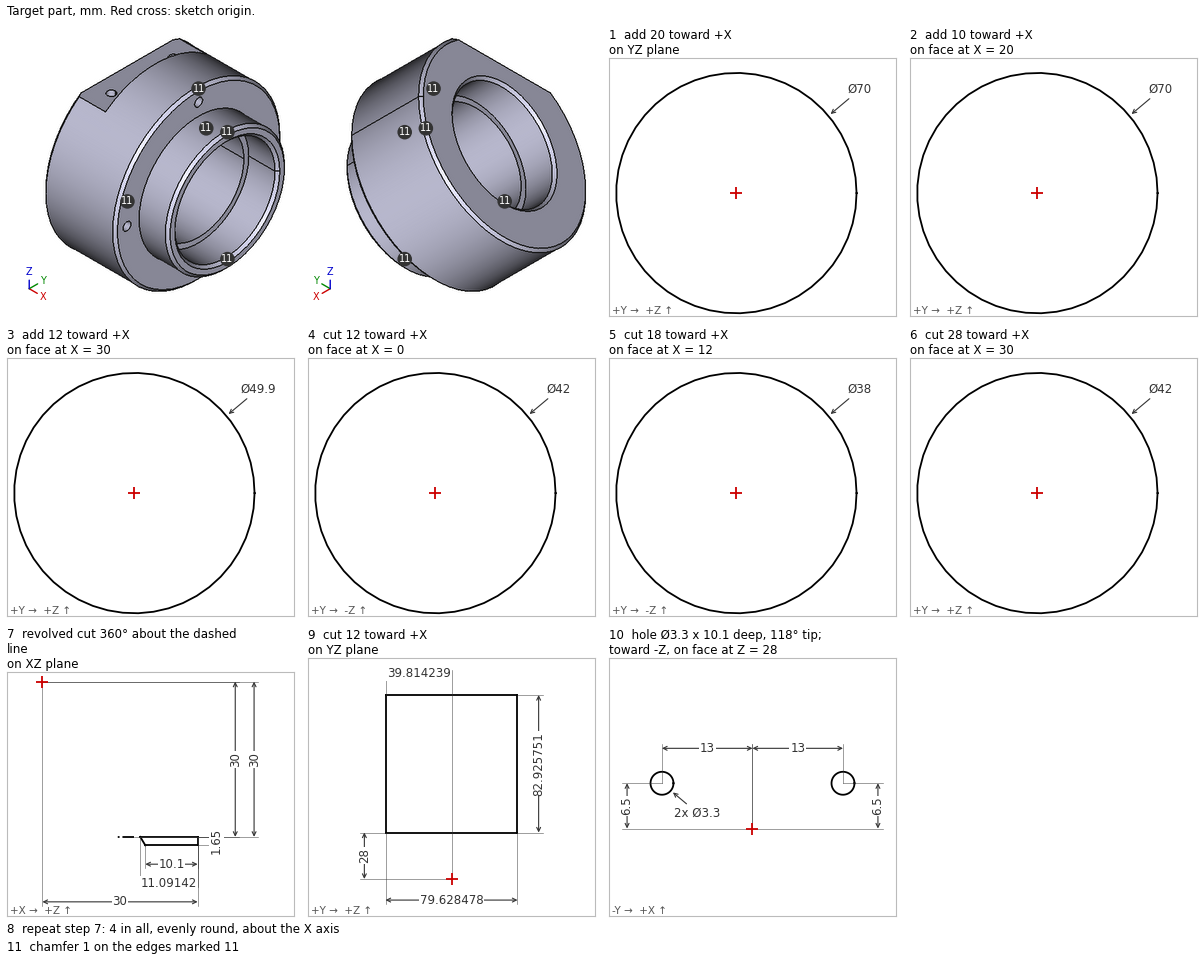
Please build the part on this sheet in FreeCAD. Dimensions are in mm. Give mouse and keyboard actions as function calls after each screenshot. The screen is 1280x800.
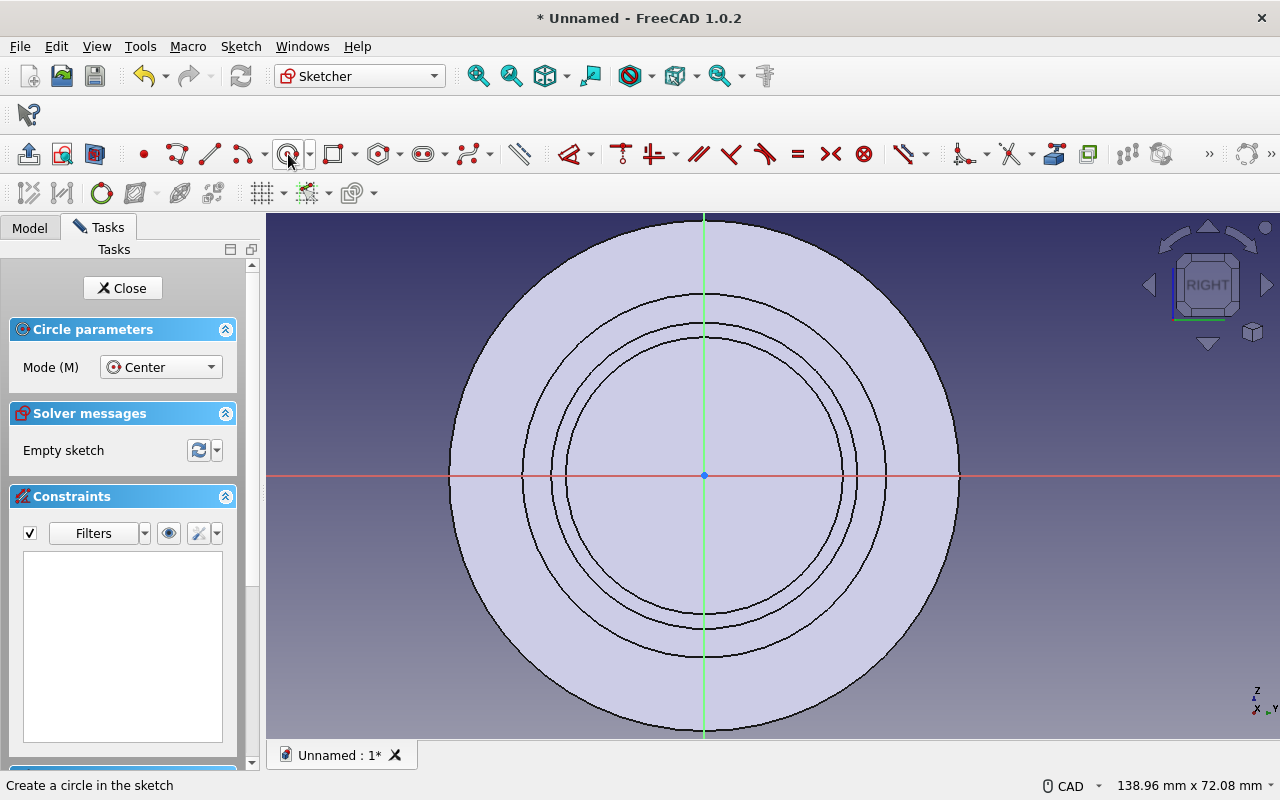
click(704, 476)
move(813, 367)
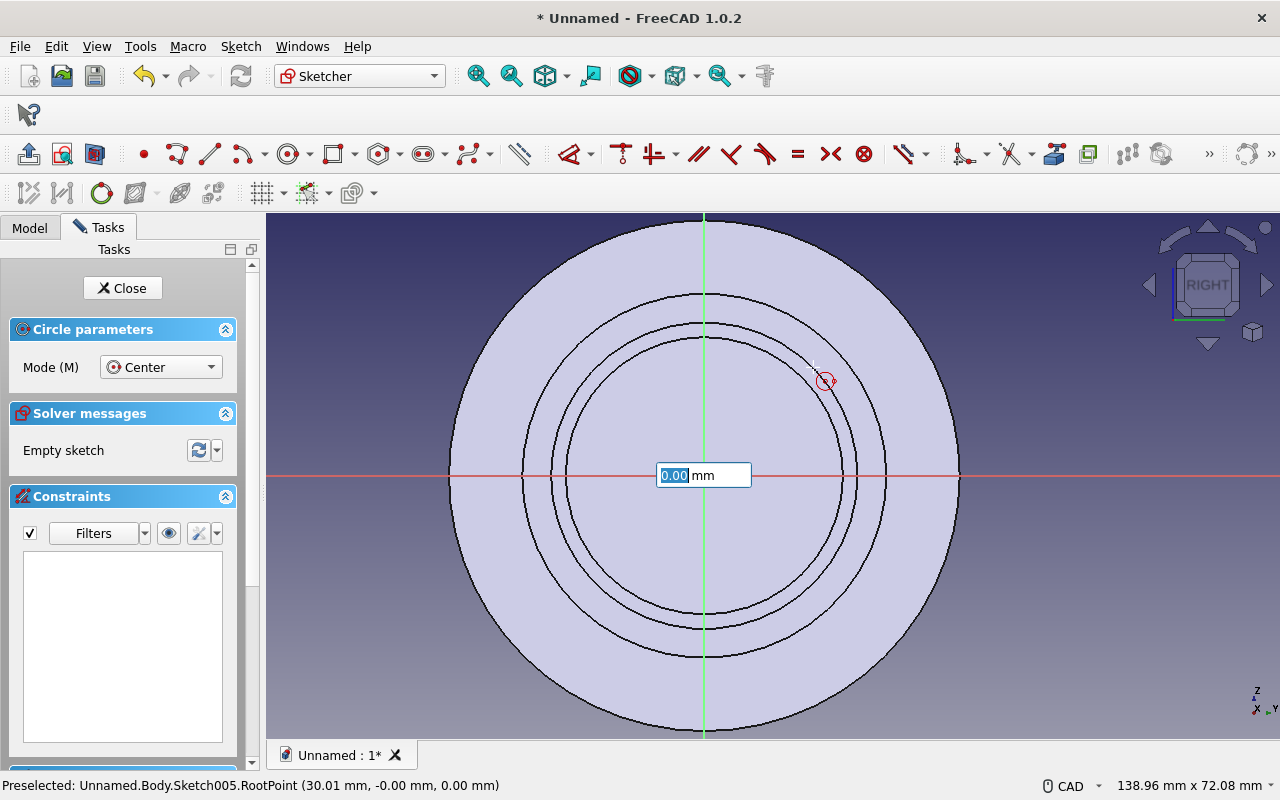
text(42)
key(Return)
key(Escape)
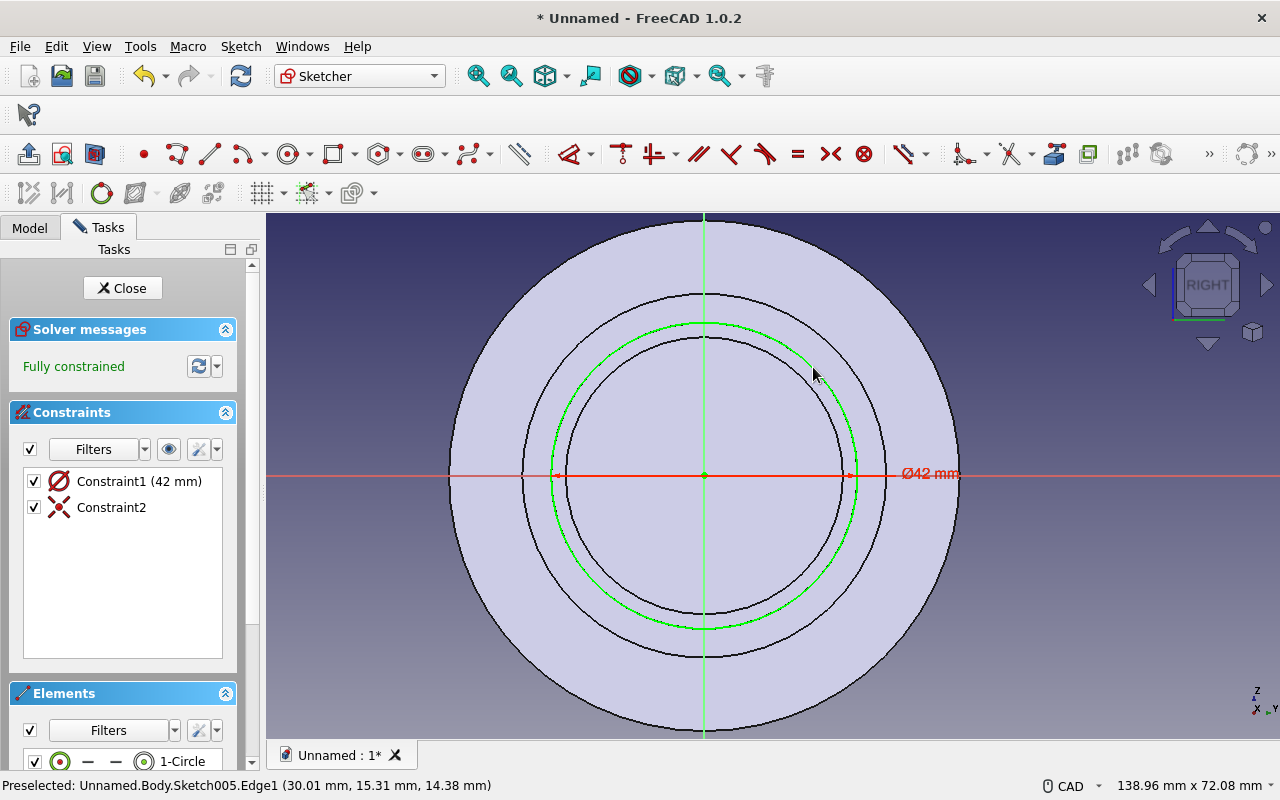
click(123, 288)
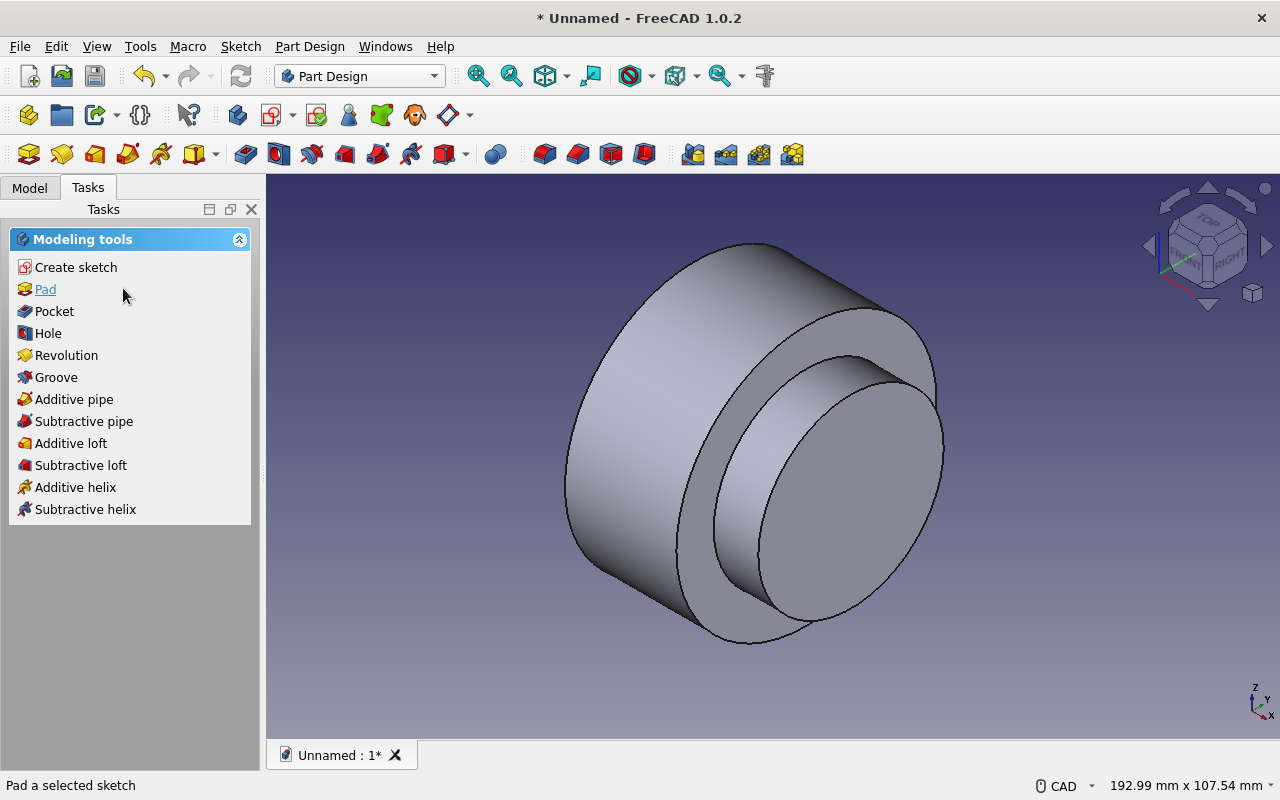
click(246, 154)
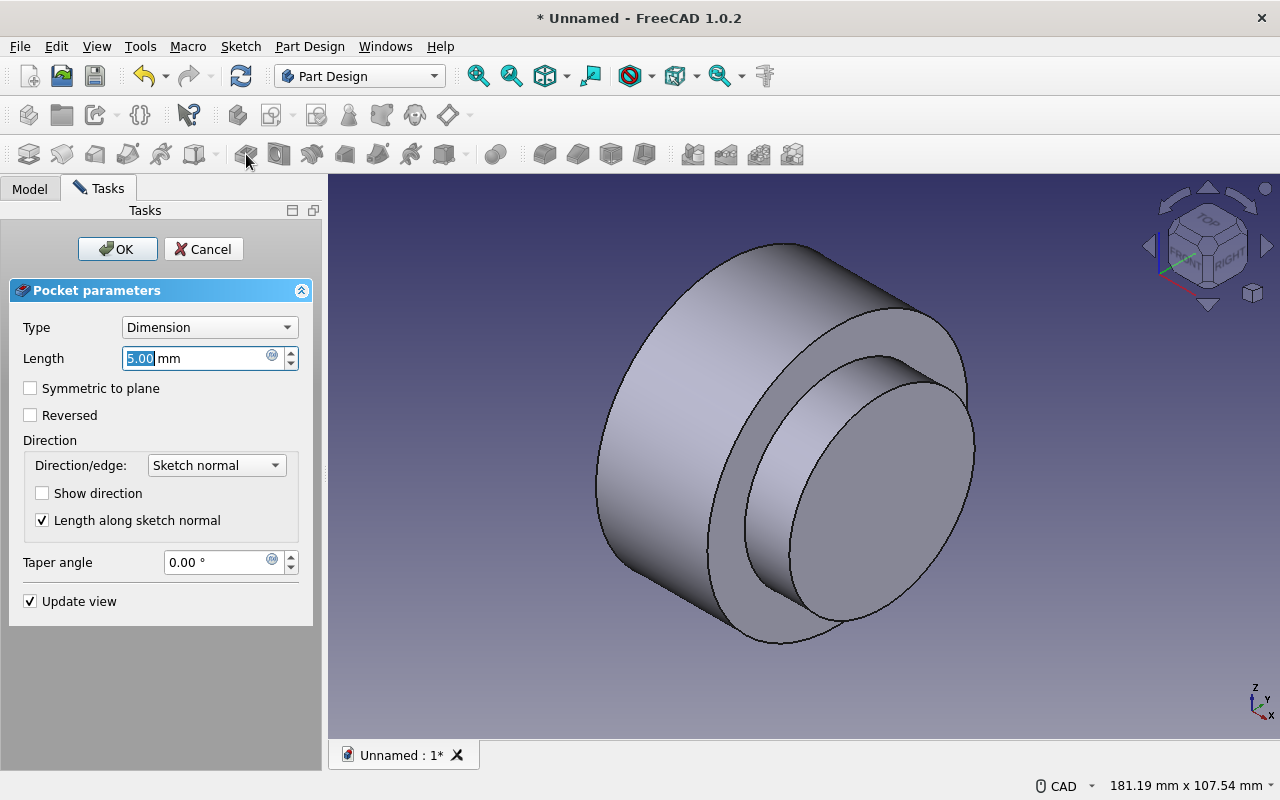
text(28)
key(Tab)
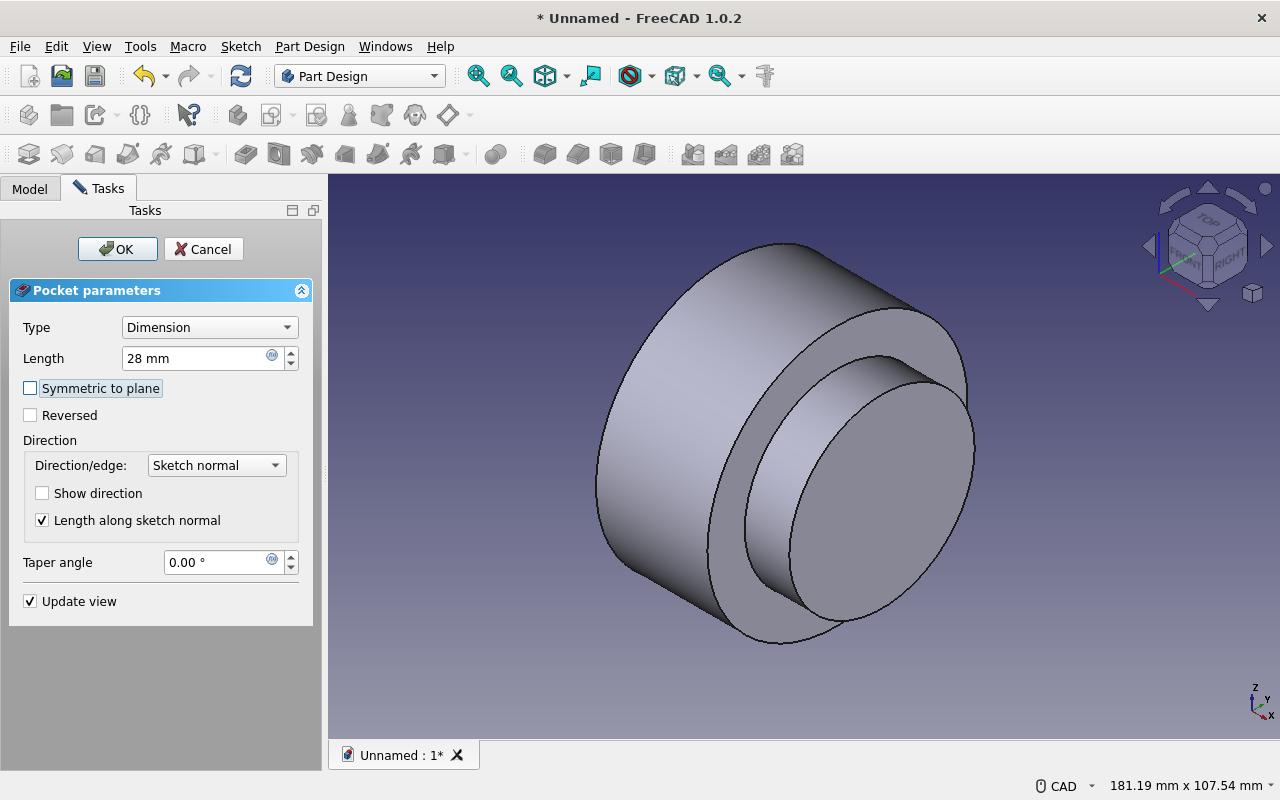
click(31, 415)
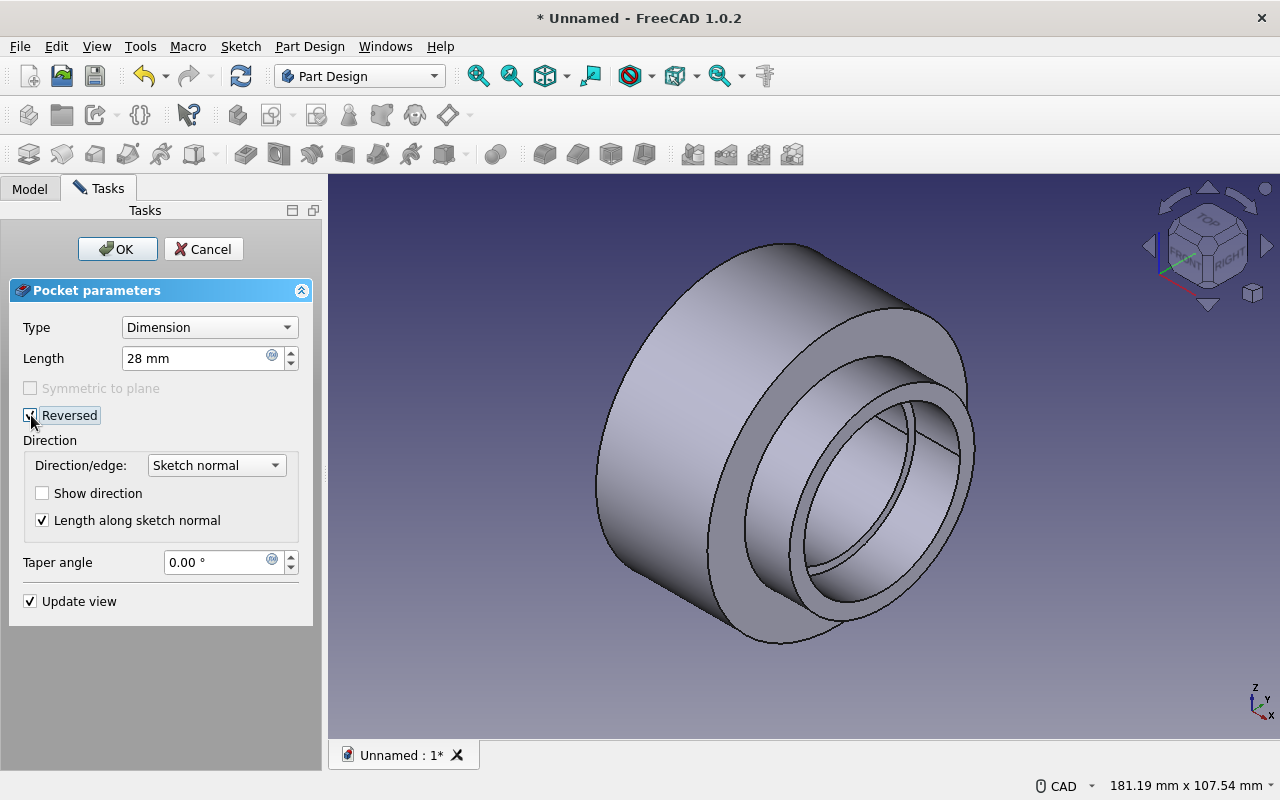
click(118, 249)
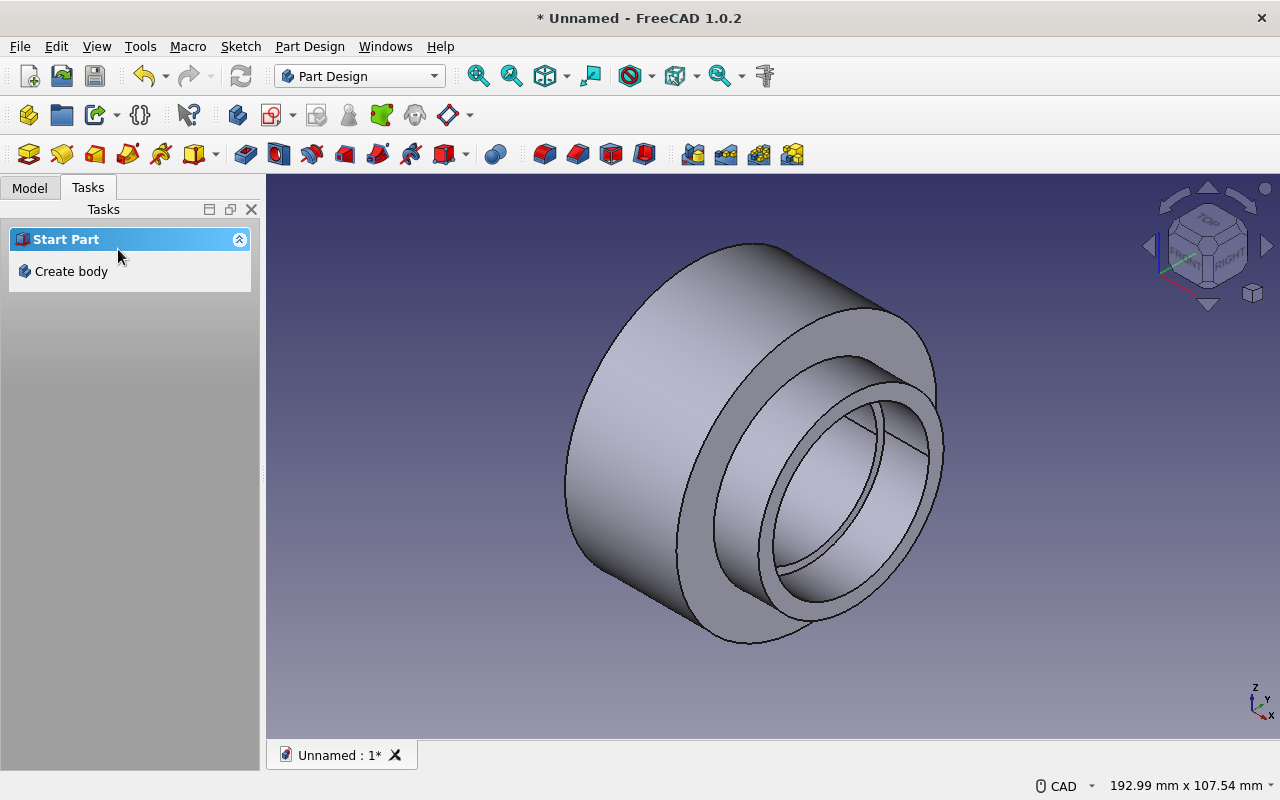
click(270, 116)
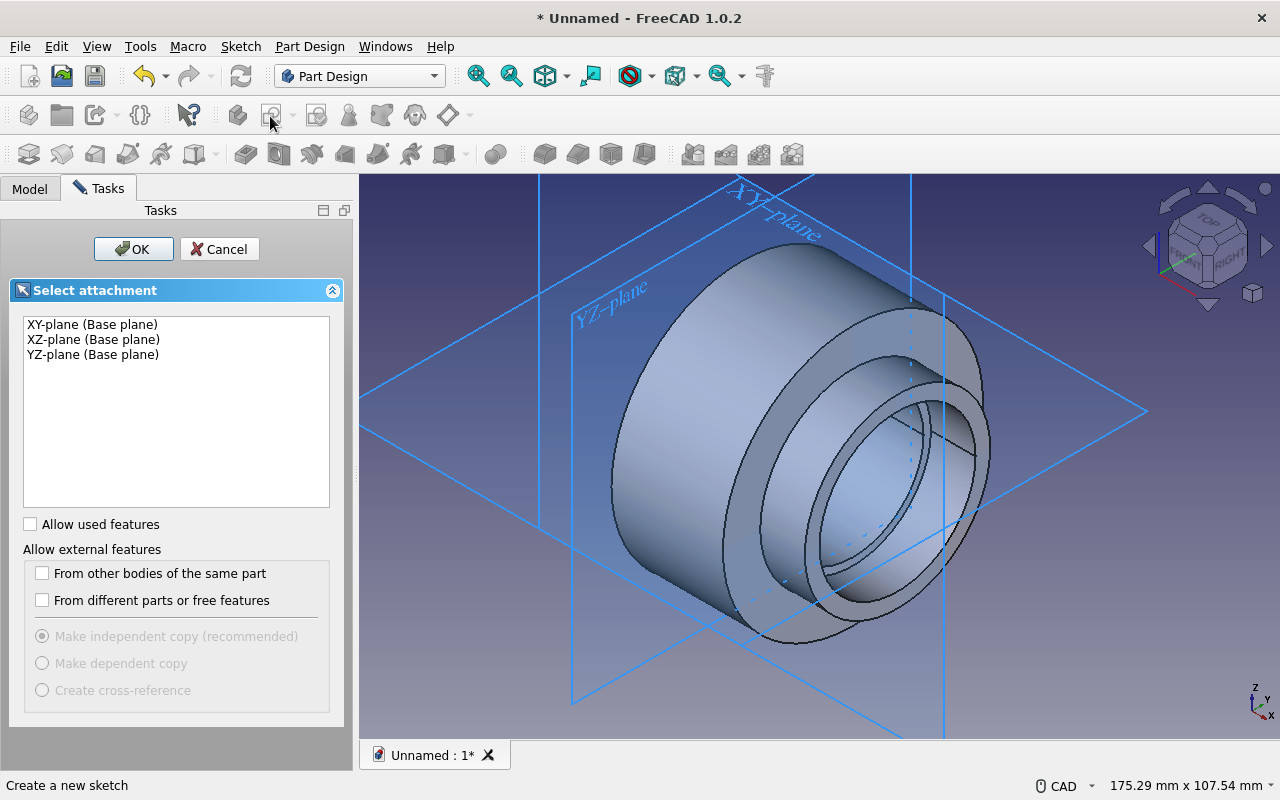
click(84, 340)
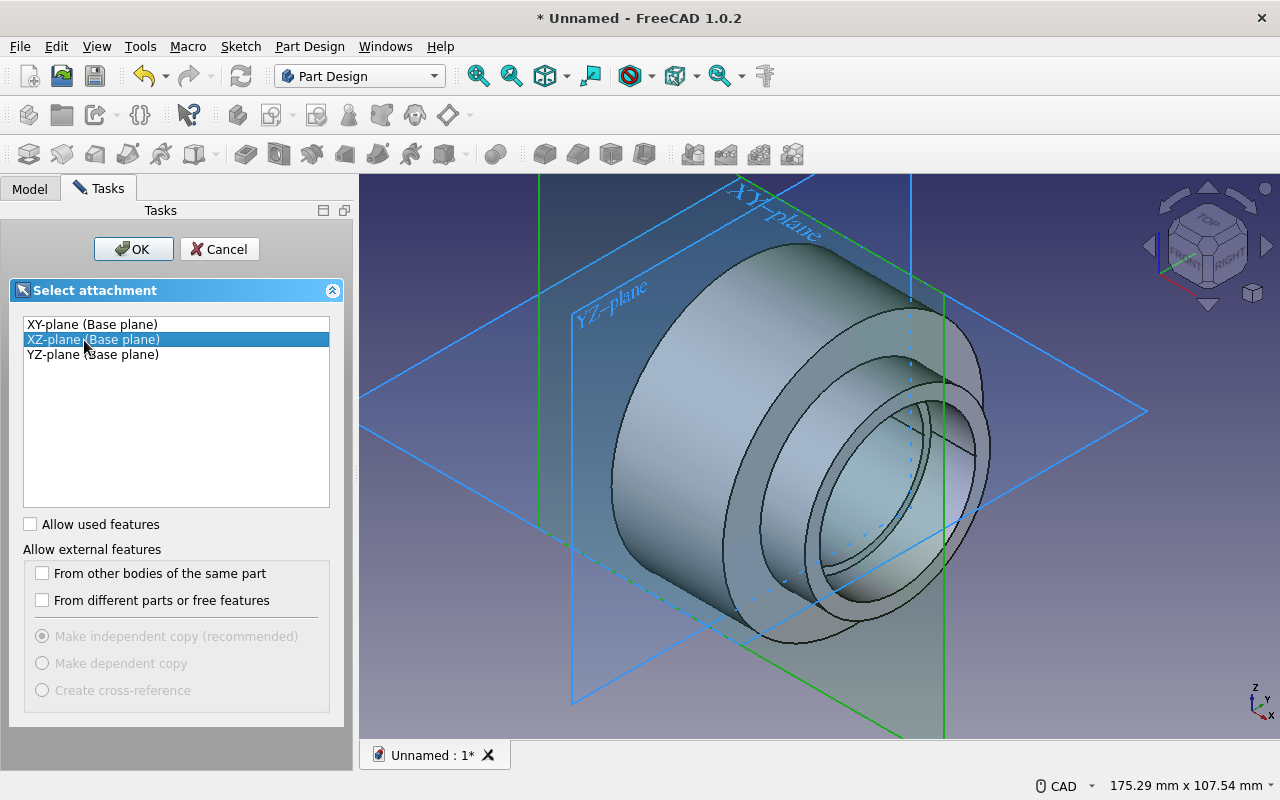
click(134, 249)